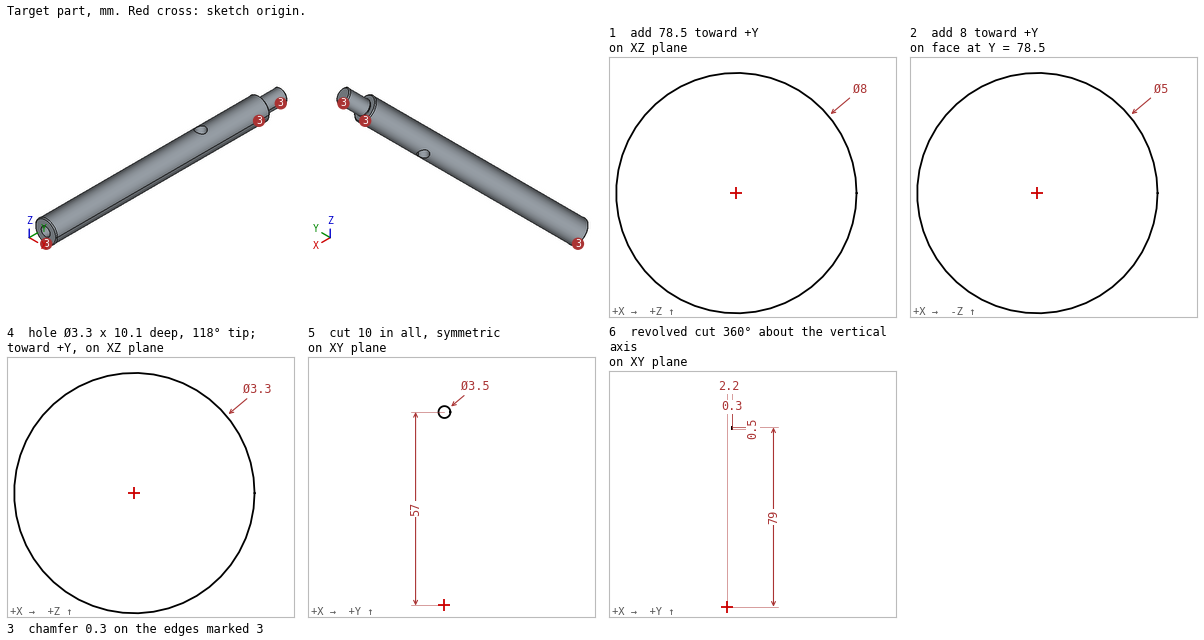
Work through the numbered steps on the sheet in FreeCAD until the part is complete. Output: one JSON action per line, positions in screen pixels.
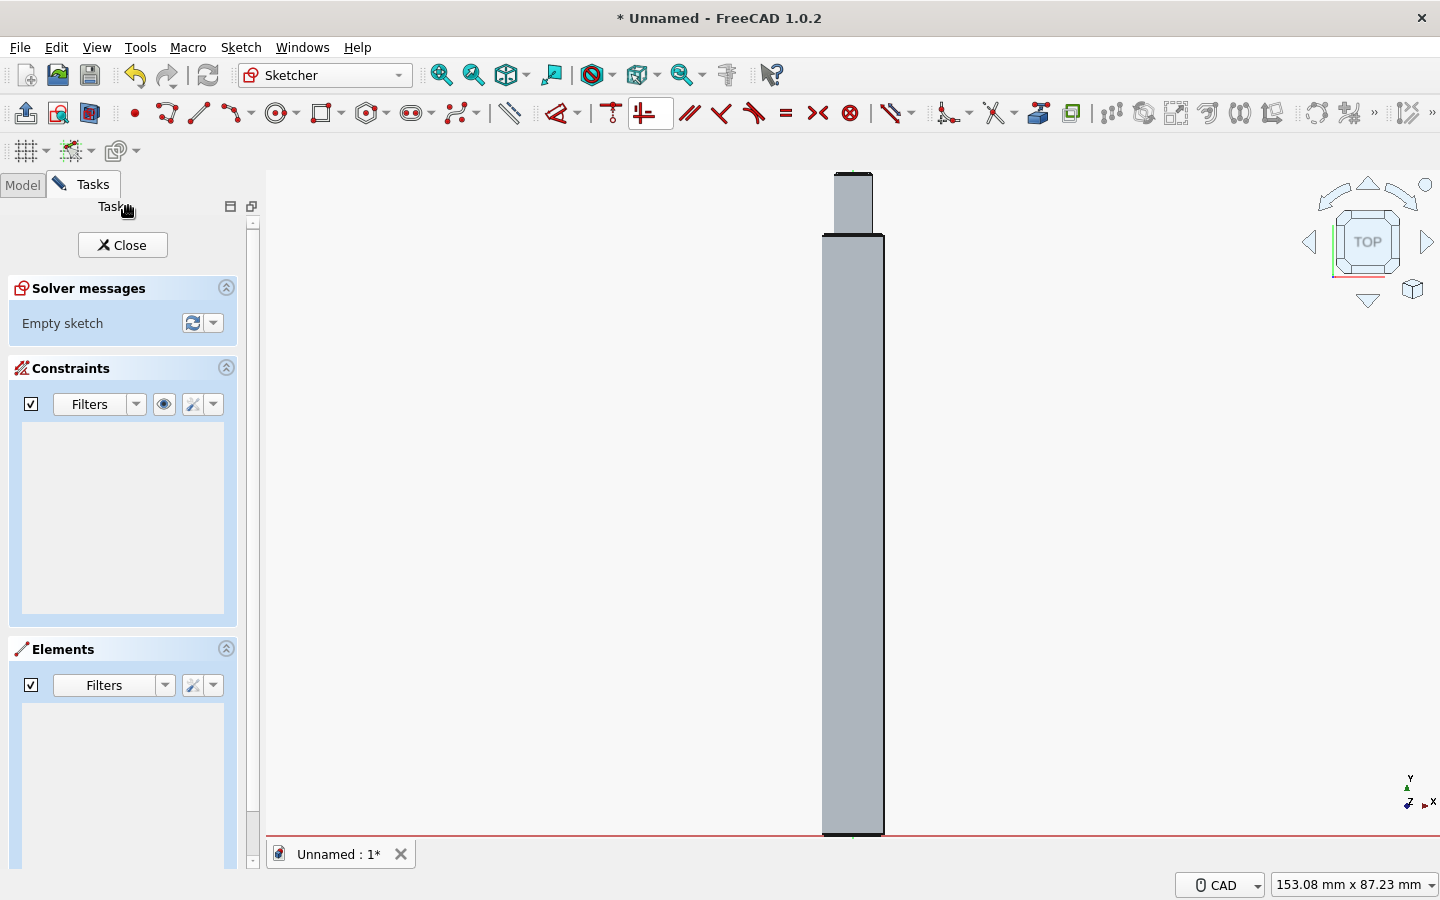
{"action": "left_click", "coordinate": [90, 114]}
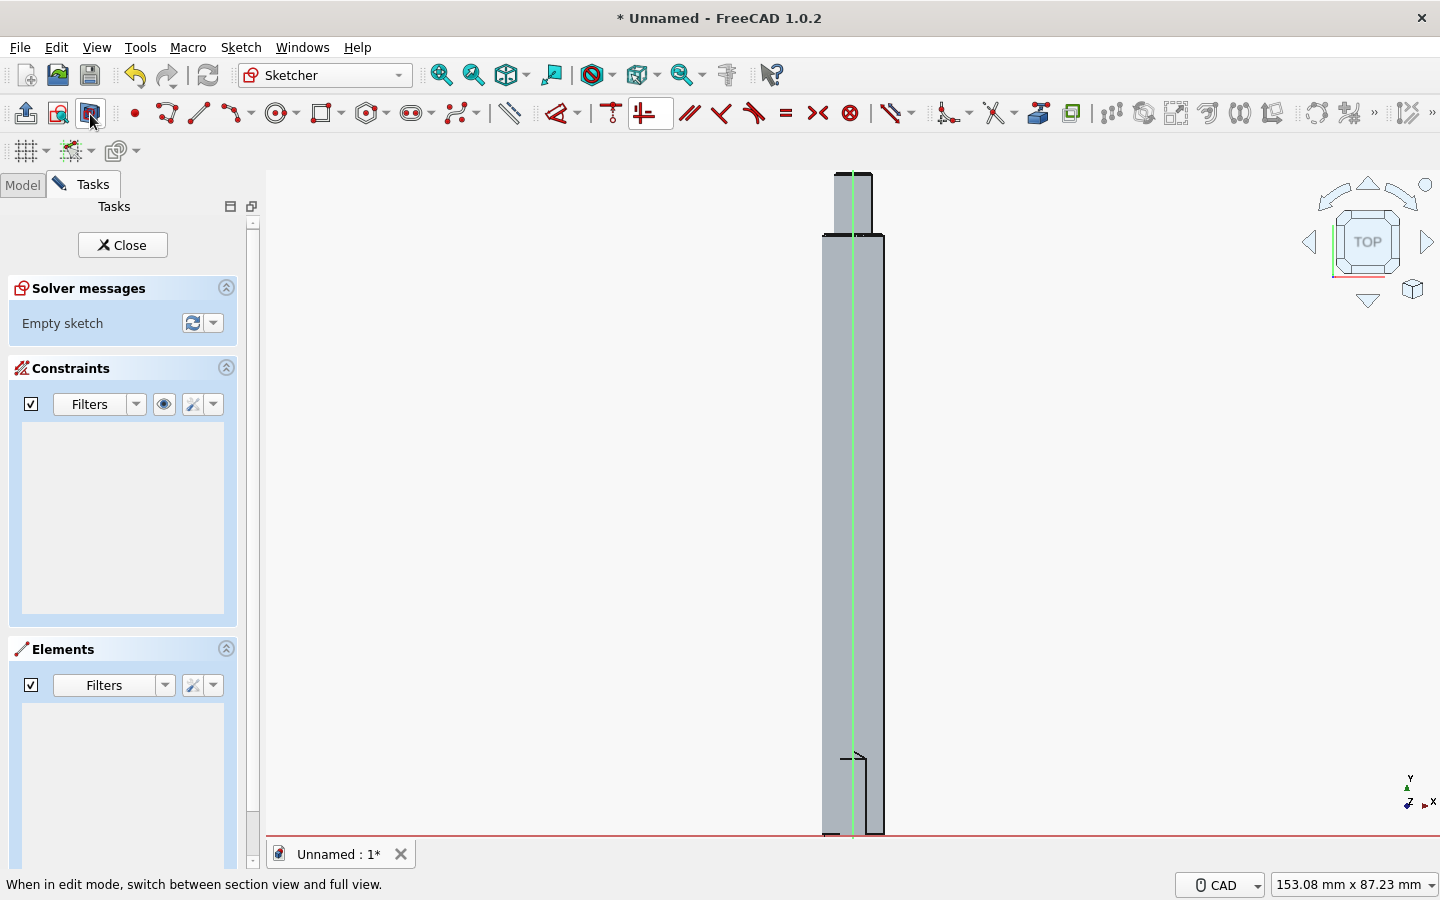
{"action": "scroll", "coordinate": [857, 392], "scroll_direction": "up", "scroll_amount": 14}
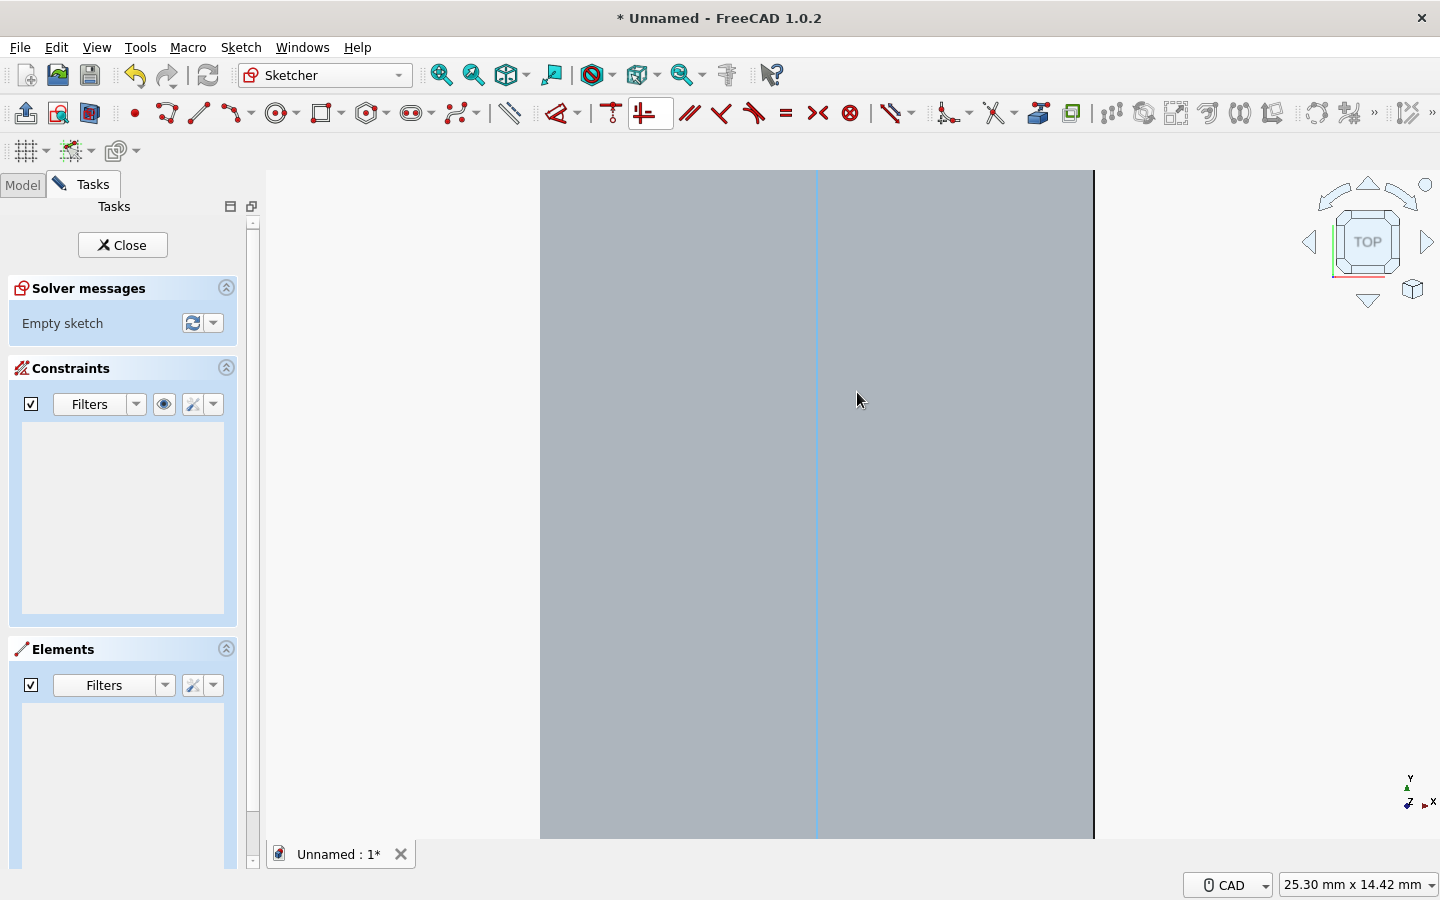
{"action": "left_click", "coordinate": [276, 114]}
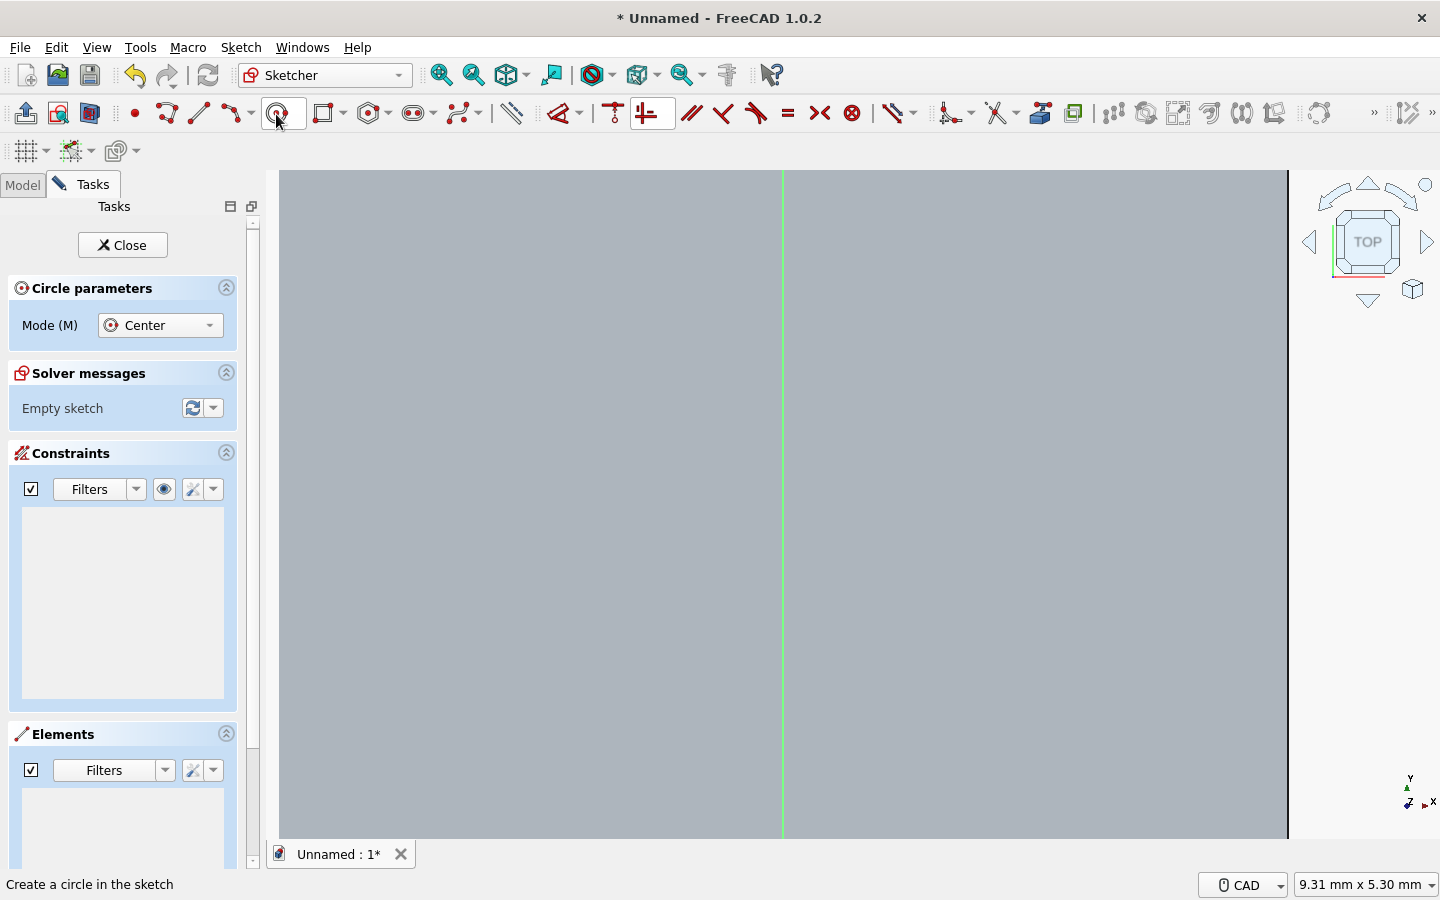
{"action": "left_click", "coordinate": [783, 503]}
{"action": "left_click", "coordinate": [940, 347]}
{"action": "key", "text": "Escape"}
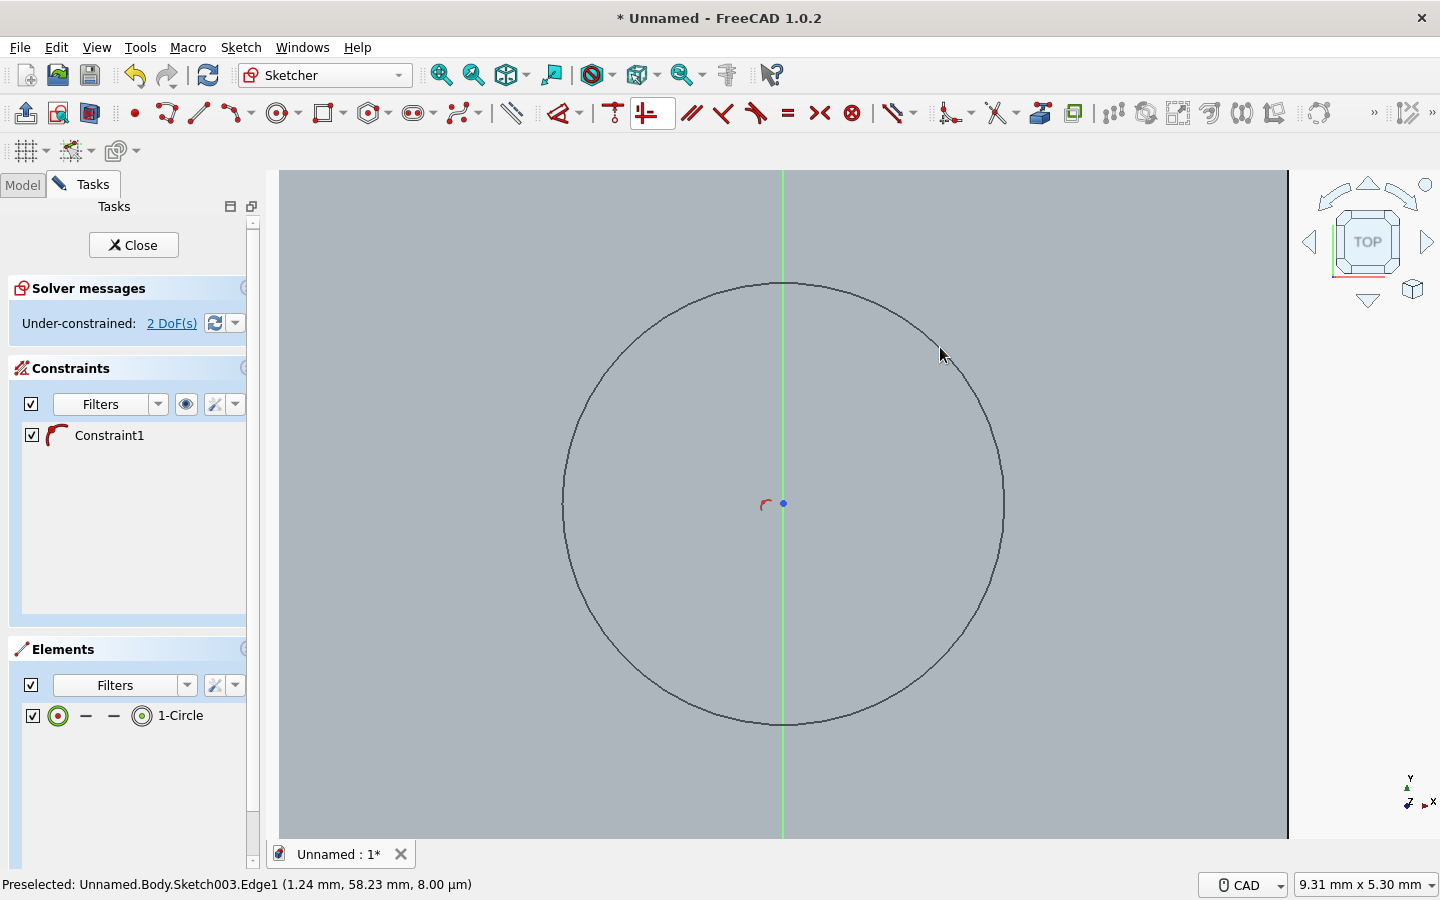
{"action": "key", "text": "d"}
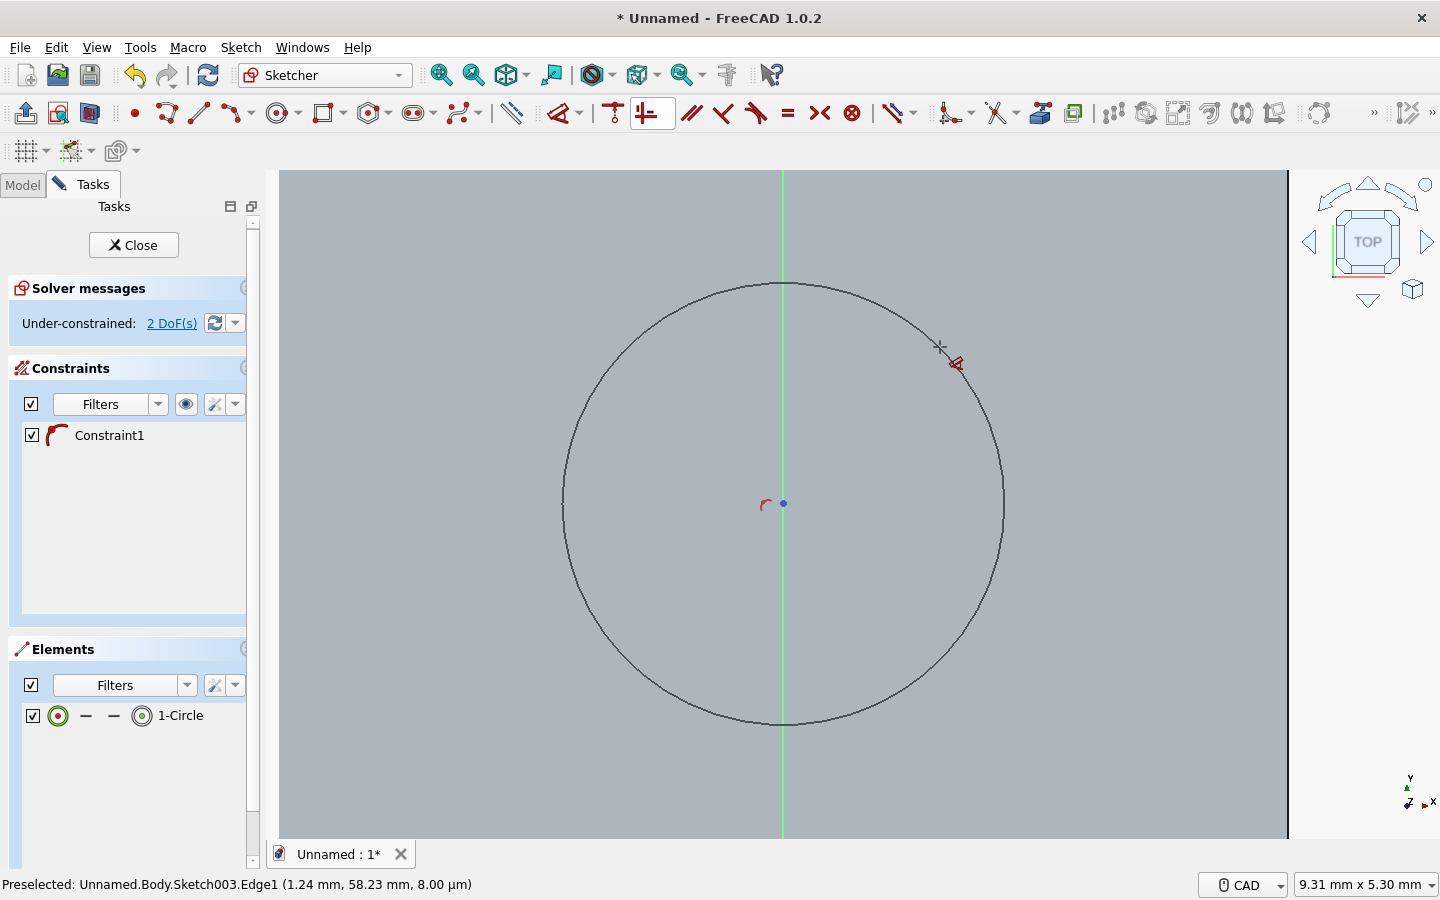
{"action": "left_click", "coordinate": [939, 347]}
{"action": "left_click", "coordinate": [962, 324]}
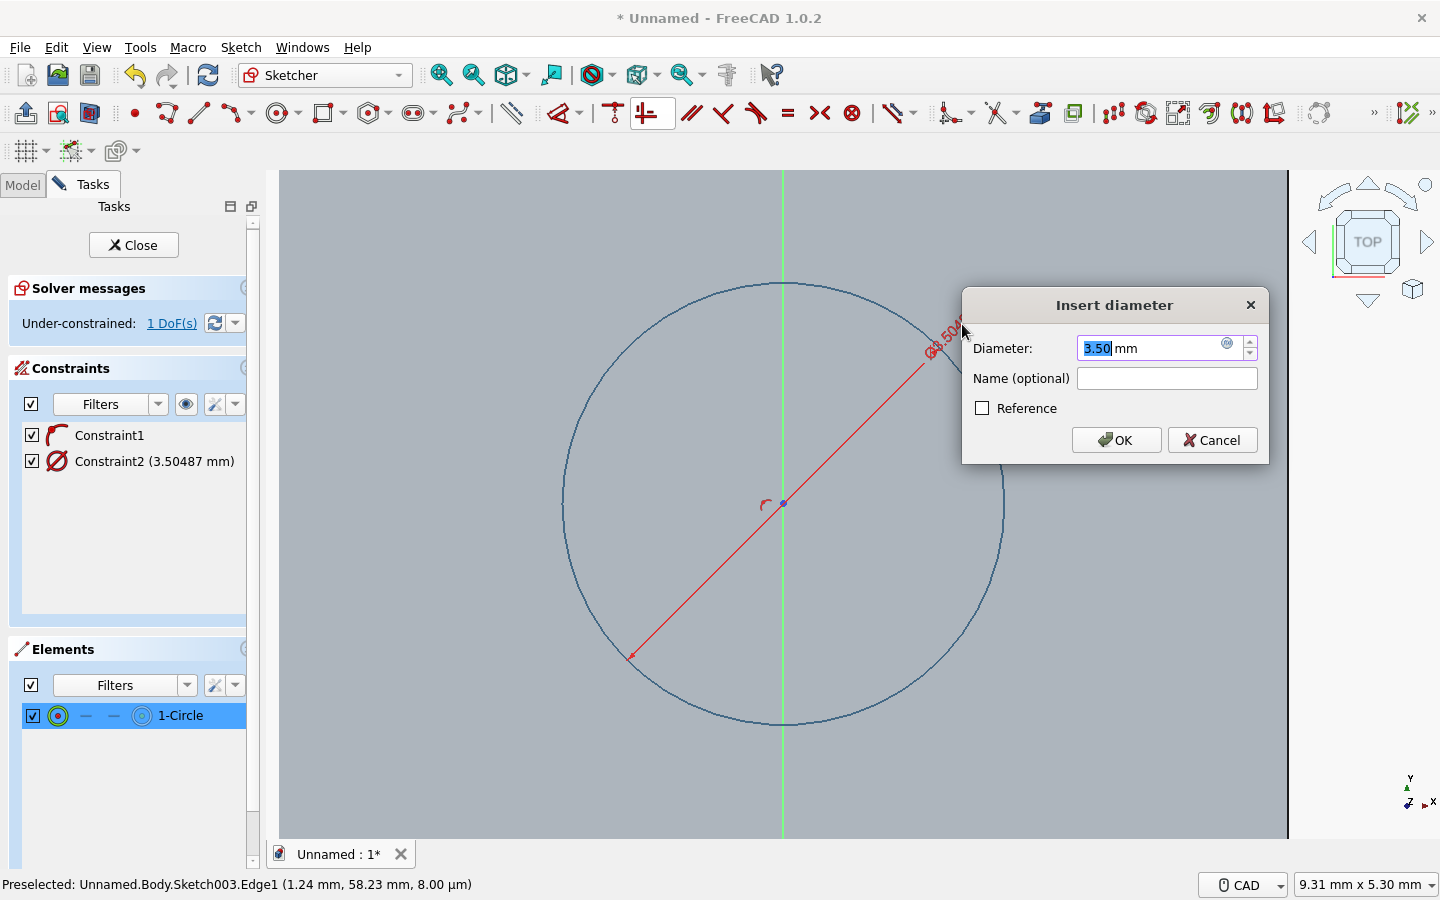
{"action": "type", "text": "3.5"}
{"action": "key", "text": "Return"}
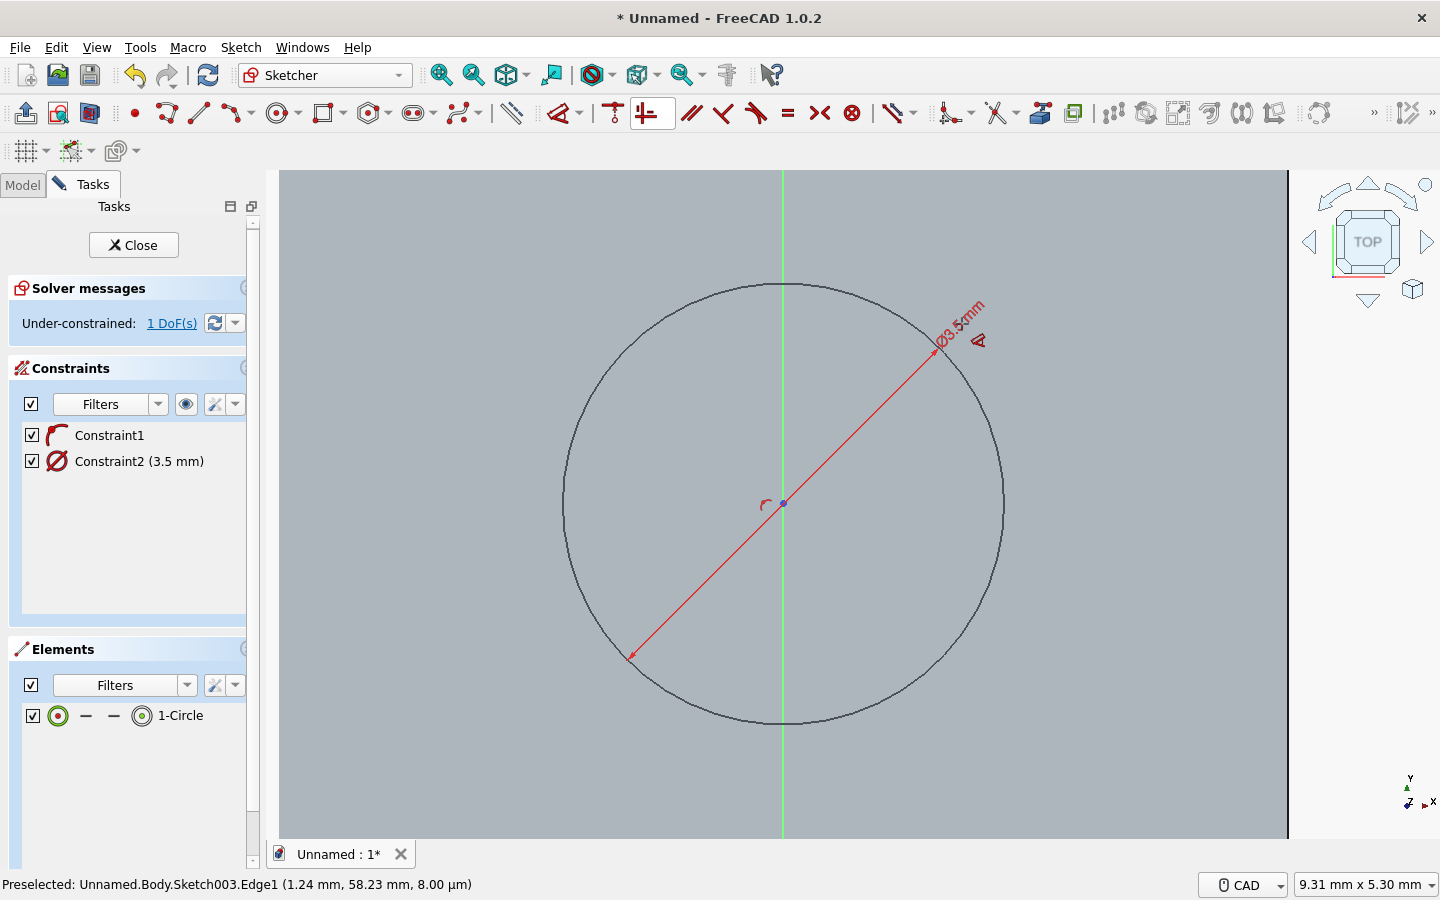
{"action": "left_click", "coordinate": [783, 504]}
{"action": "left_click", "coordinate": [817, 658]}